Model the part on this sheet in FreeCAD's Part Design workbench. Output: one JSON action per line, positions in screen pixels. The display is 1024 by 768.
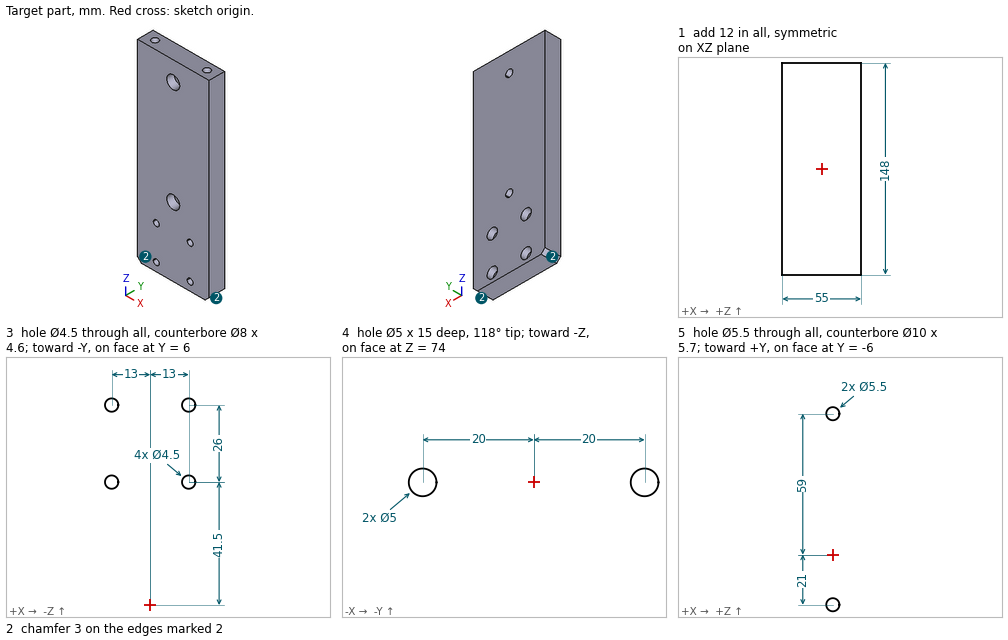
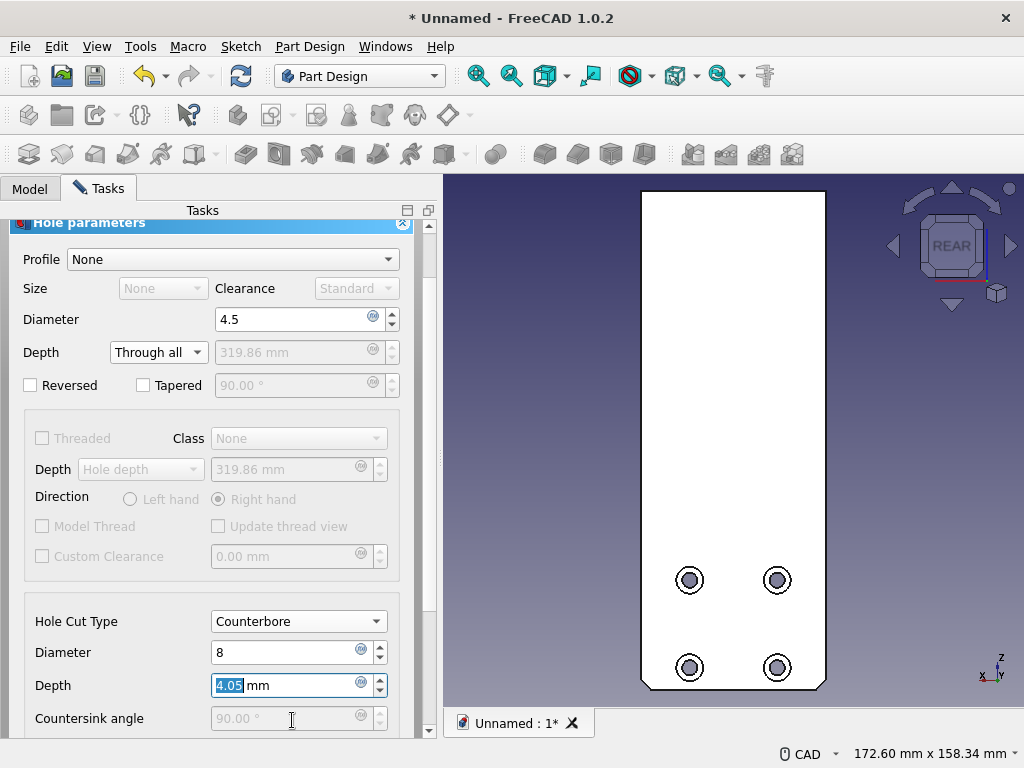
{"action": "type", "text": "4.6"}
{"action": "key", "text": "Tab"}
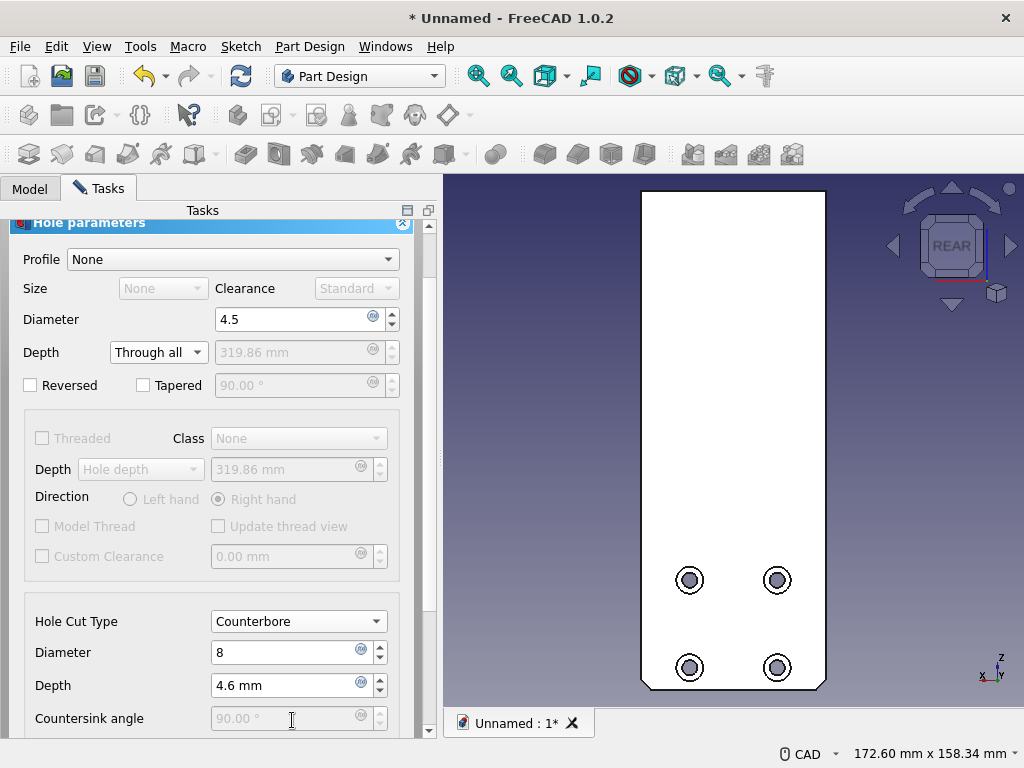
{"action": "scroll", "coordinate": [429, 479], "scroll_direction": "up", "scroll_amount": 2}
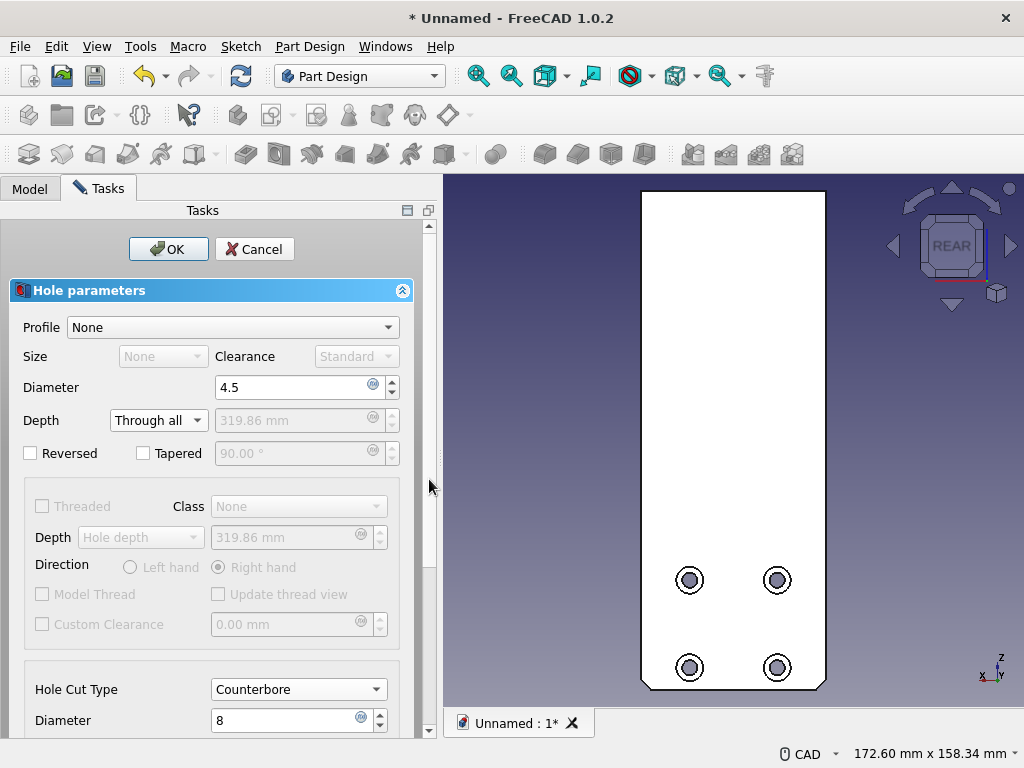
{"action": "left_click", "coordinate": [169, 249]}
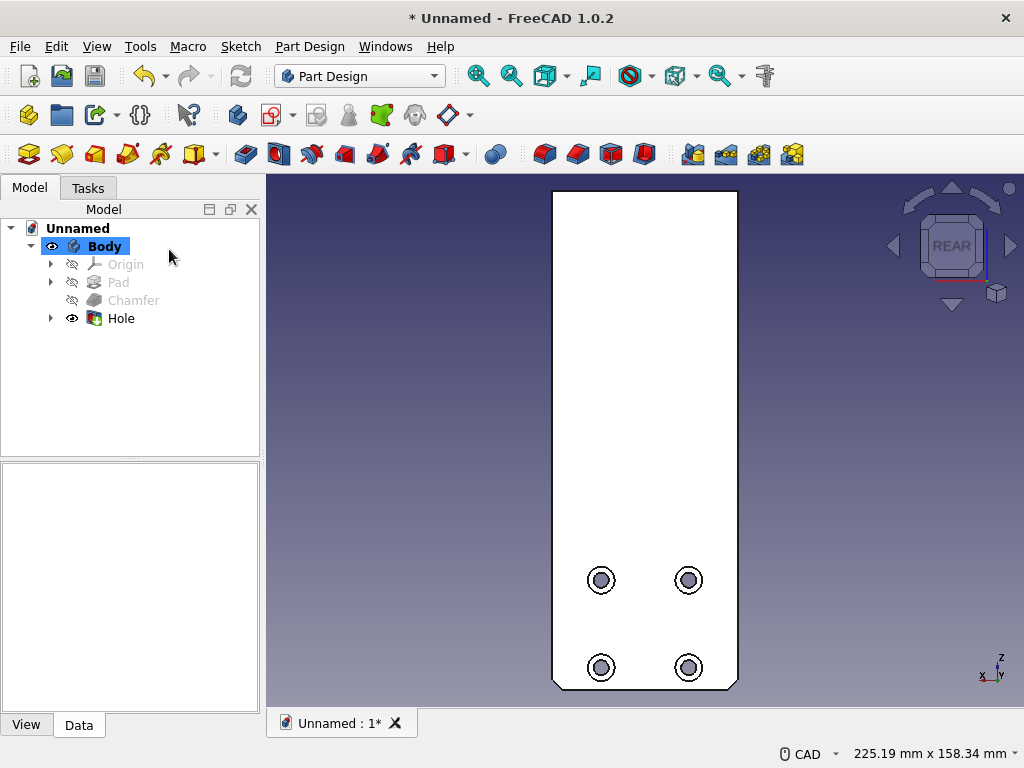
{"action": "key", "text": "0"}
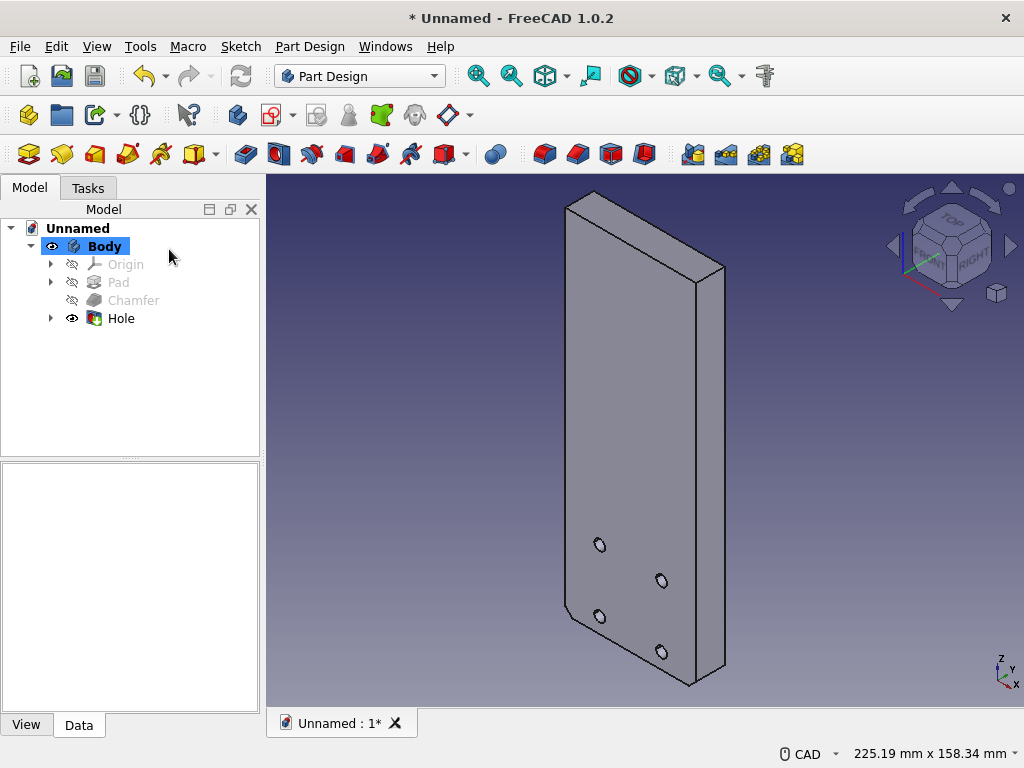
{"action": "left_click", "coordinate": [682, 258]}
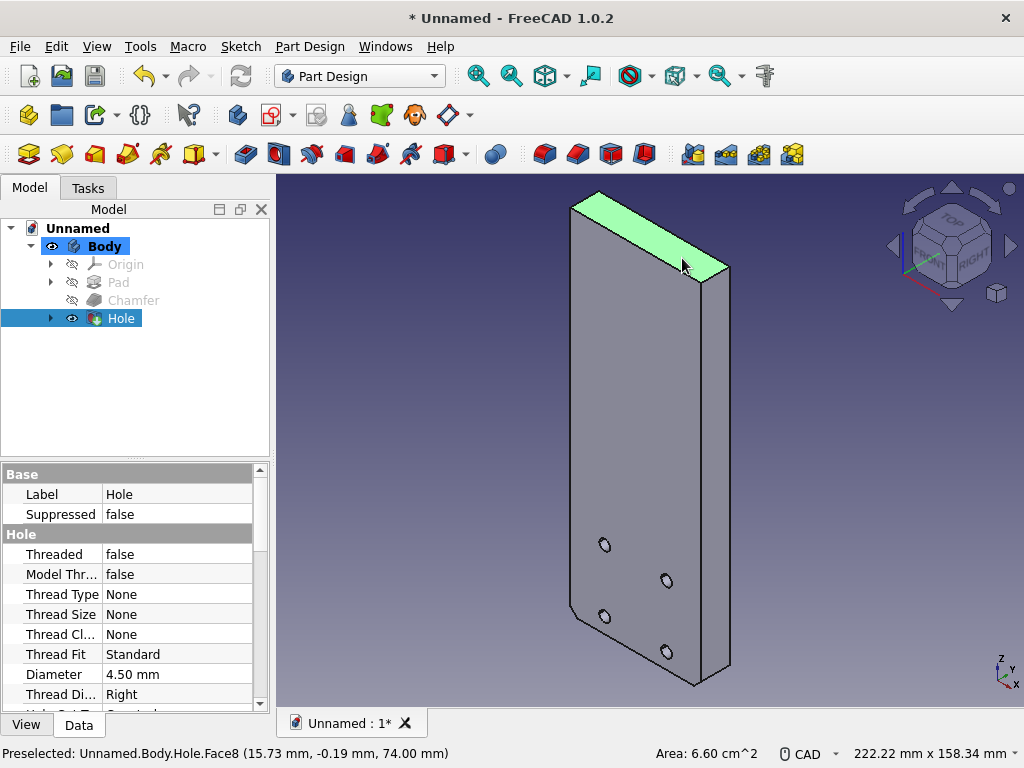
{"action": "left_click", "coordinate": [270, 116]}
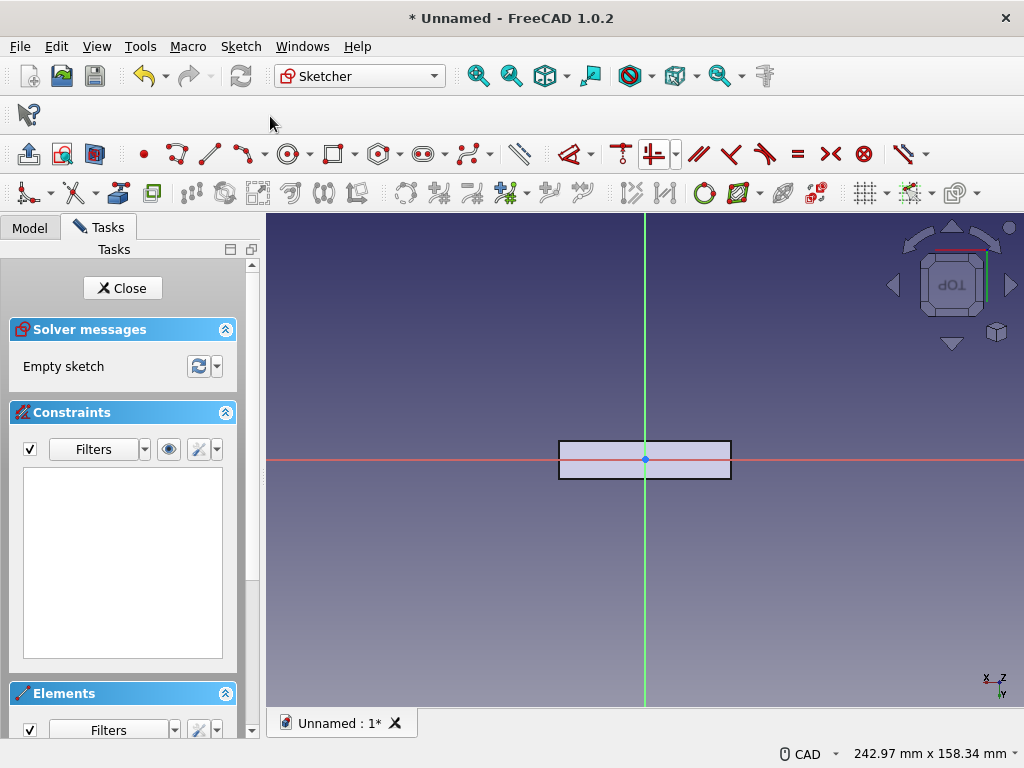
{"action": "scroll", "coordinate": [685, 460], "scroll_direction": "up", "scroll_amount": 5}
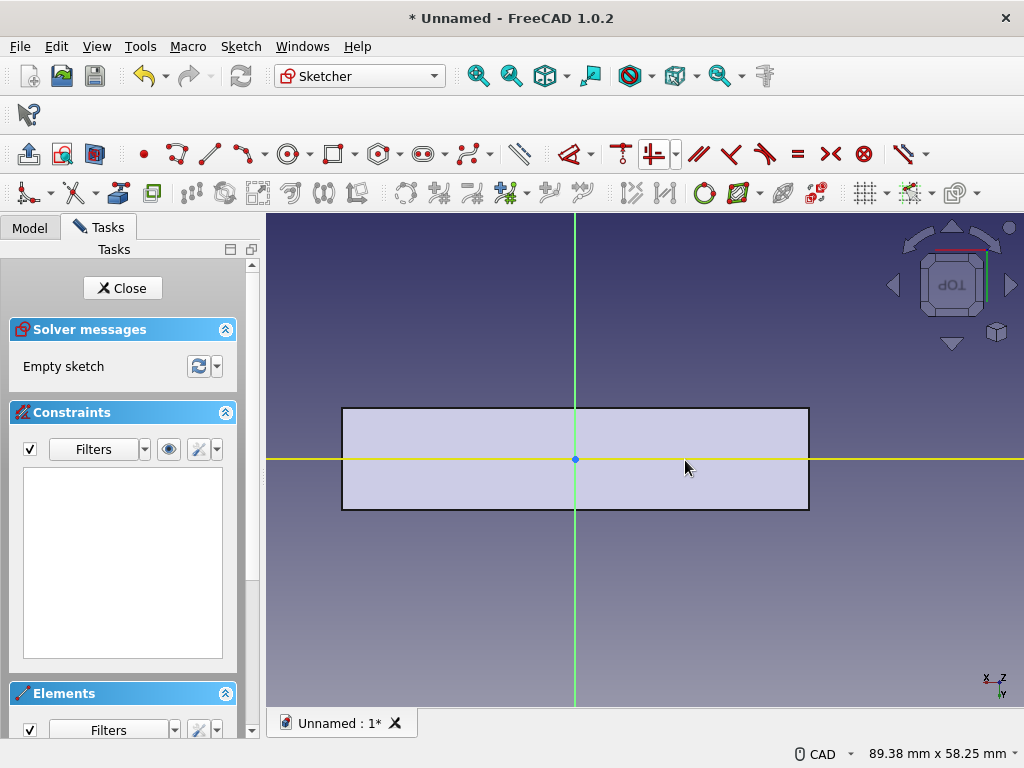
{"action": "left_click", "coordinate": [288, 154]}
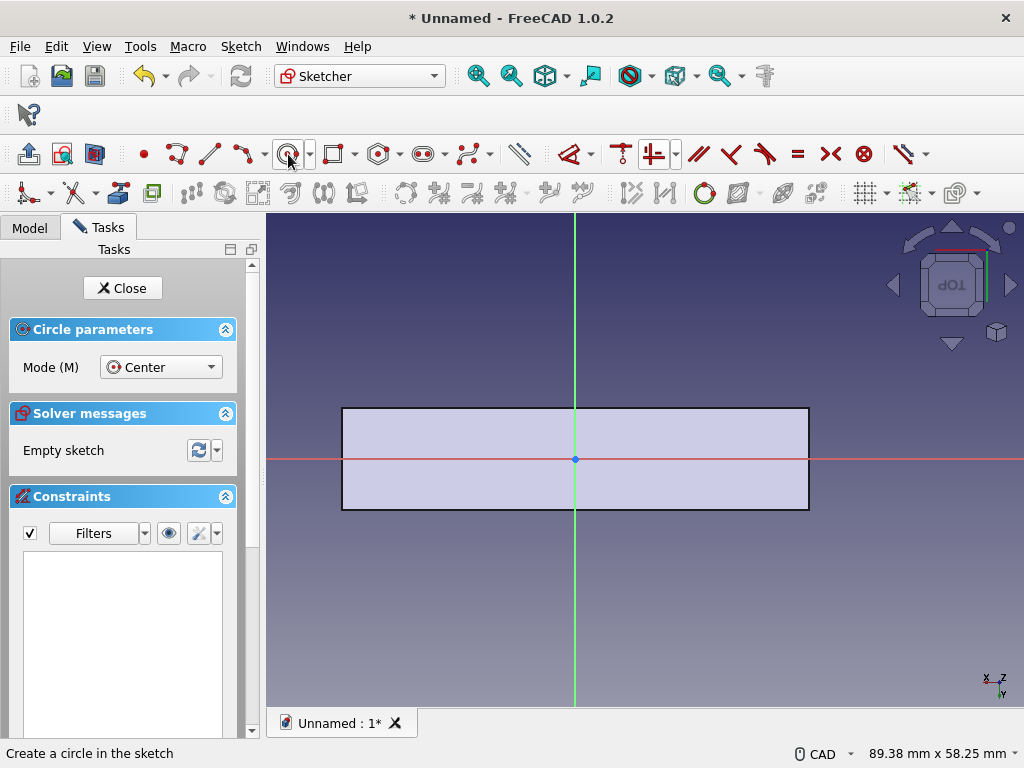
{"action": "left_click", "coordinate": [406, 459]}
{"action": "mouse_move", "coordinate": [421, 444]}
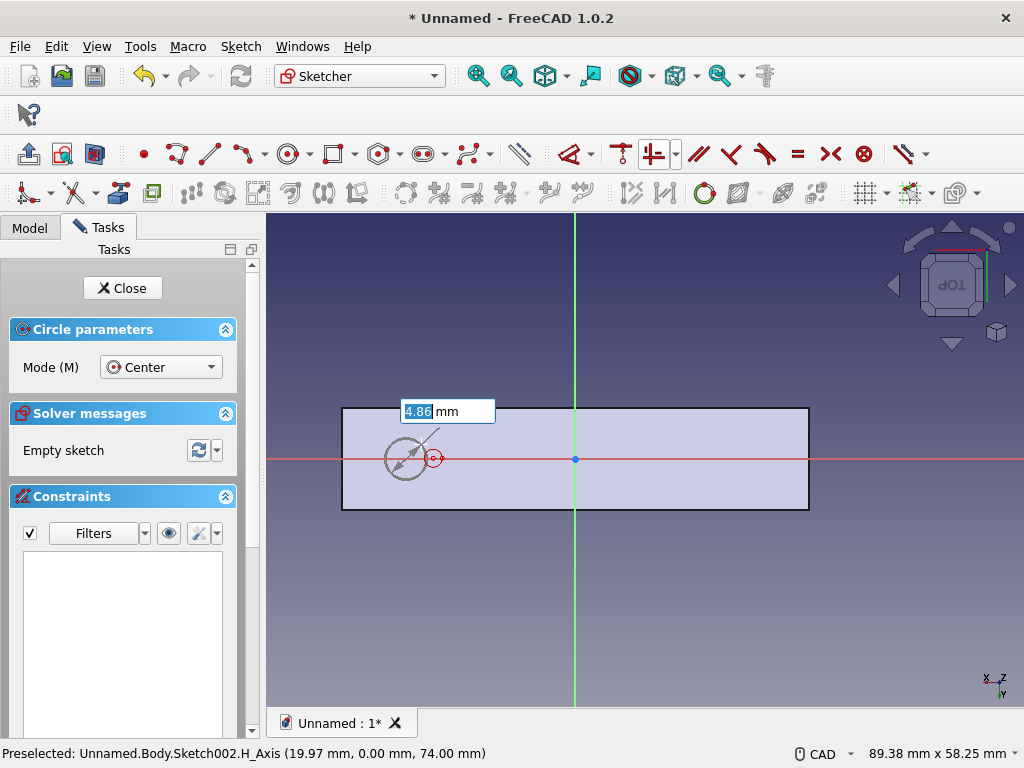
{"action": "type", "text": "5"}
{"action": "key", "text": "Return"}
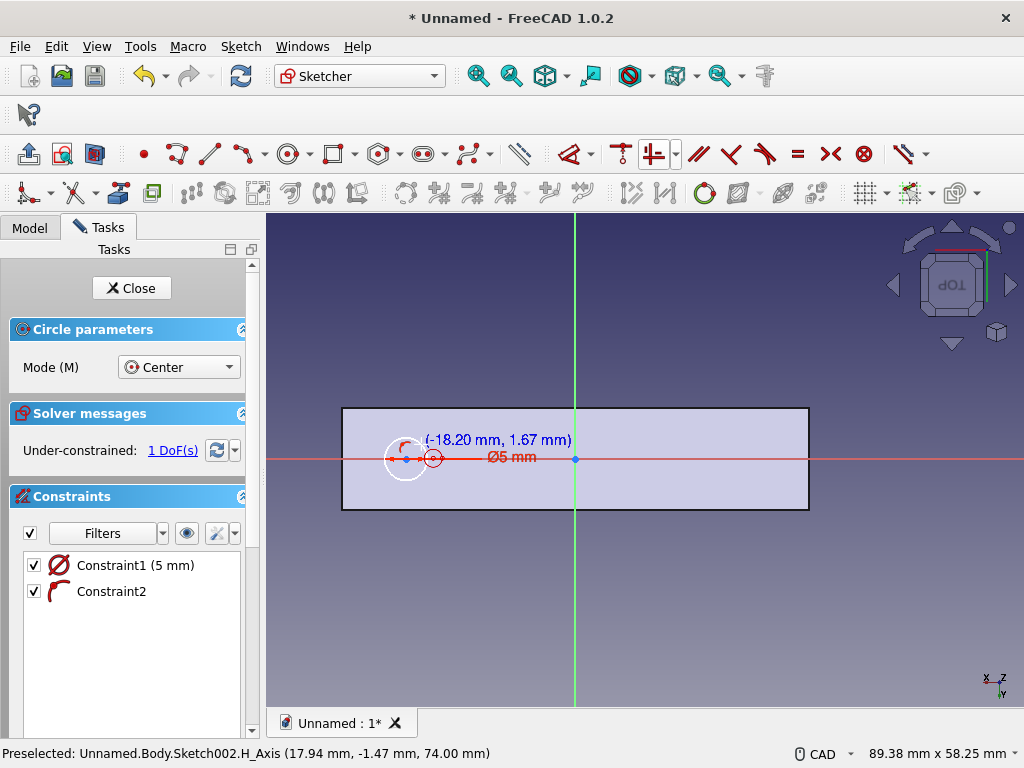
{"action": "left_click", "coordinate": [745, 459]}
{"action": "mouse_move", "coordinate": [760, 444]}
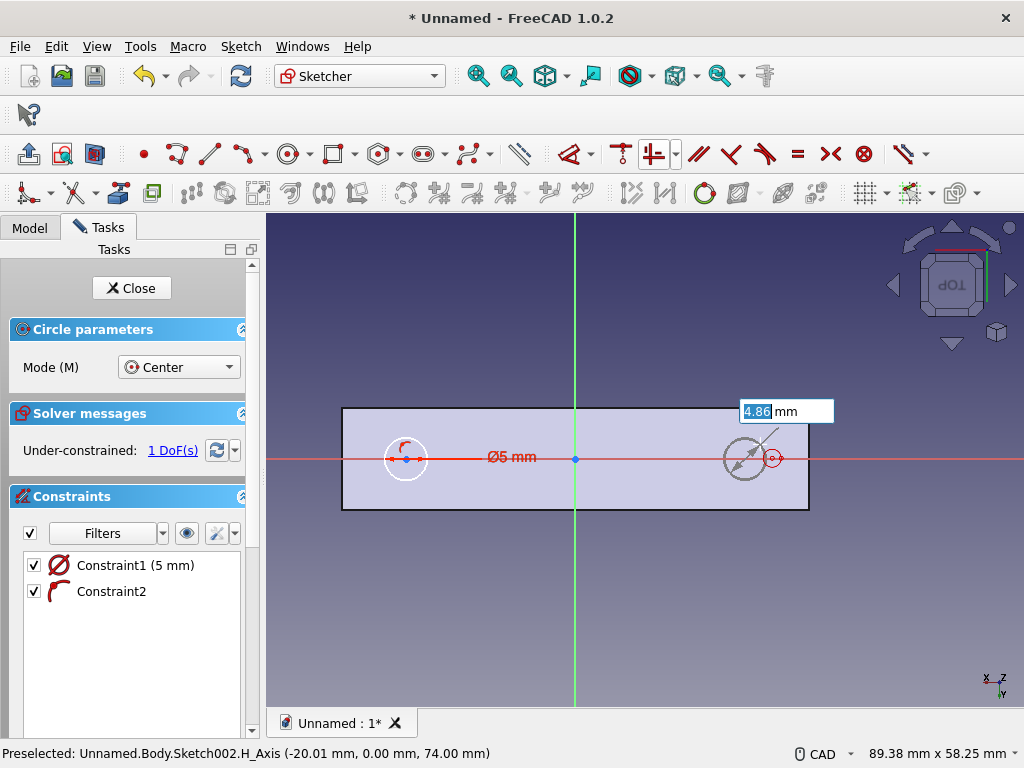
{"action": "type", "text": "5"}
{"action": "key", "text": "Return"}
{"action": "key", "text": "Escape"}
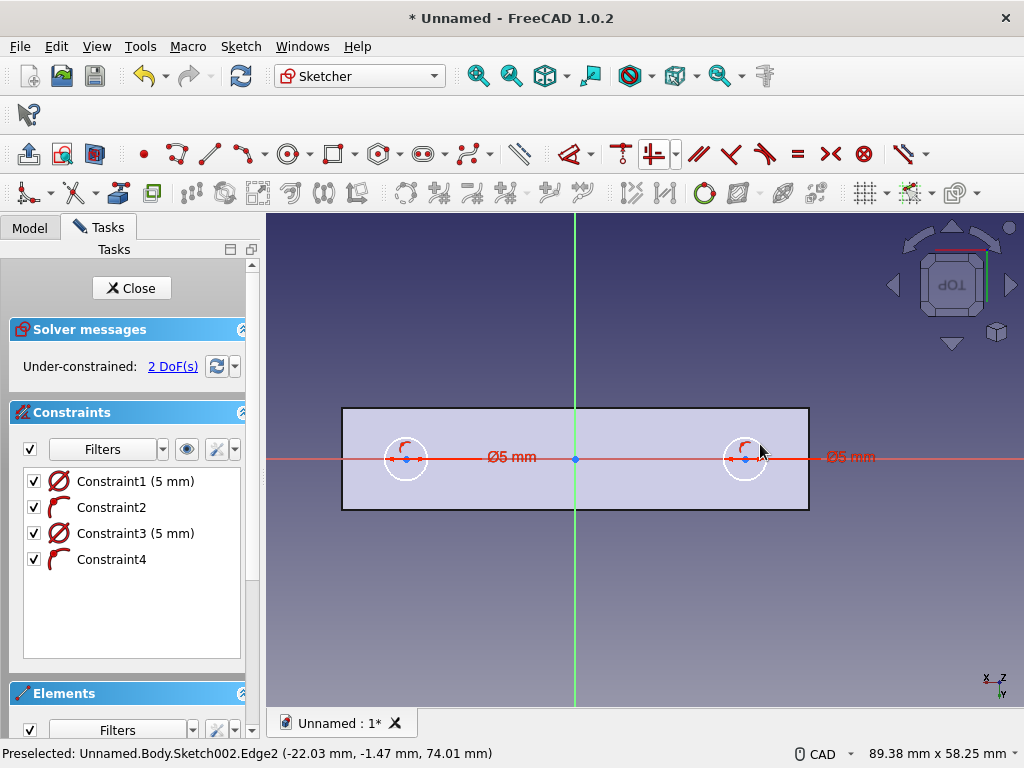
{"action": "key", "text": "d"}